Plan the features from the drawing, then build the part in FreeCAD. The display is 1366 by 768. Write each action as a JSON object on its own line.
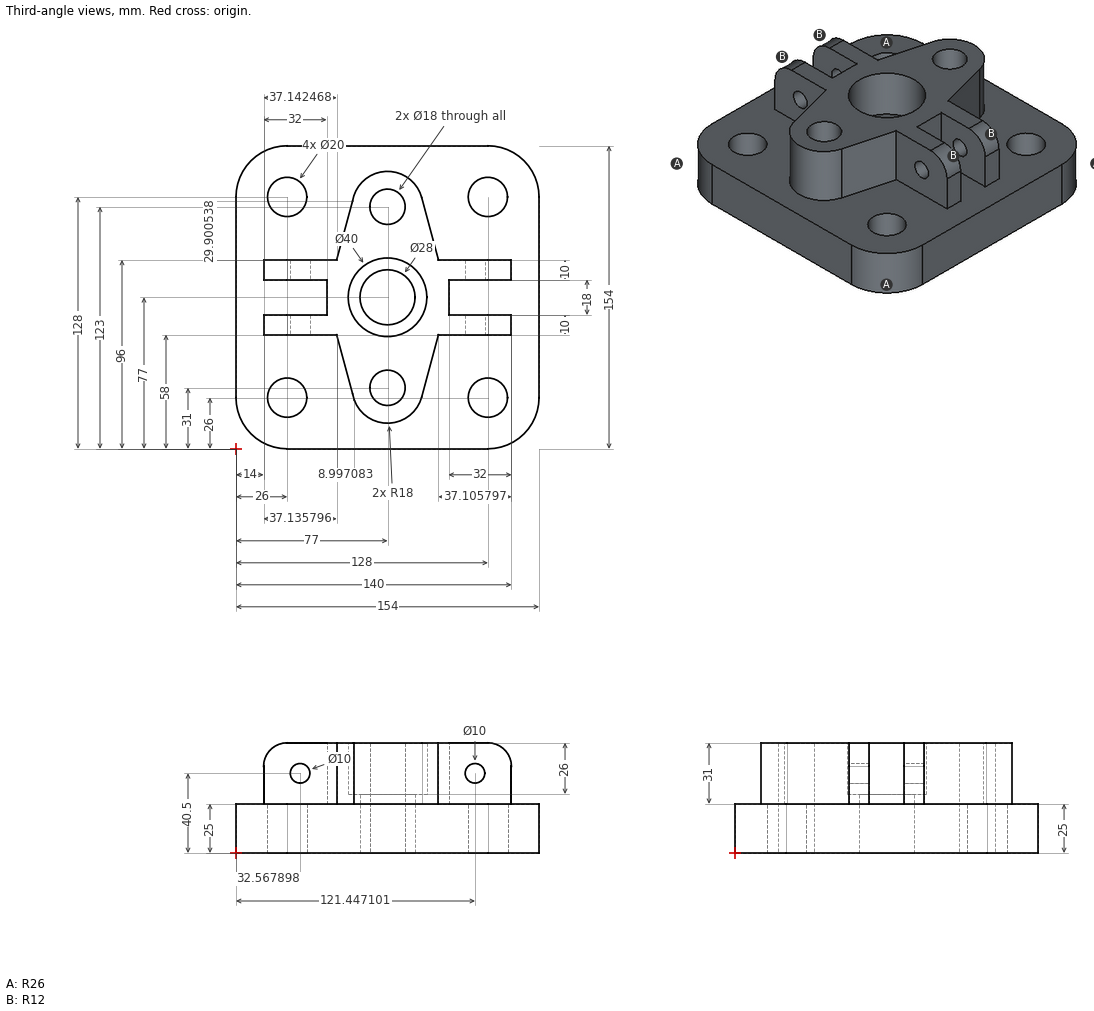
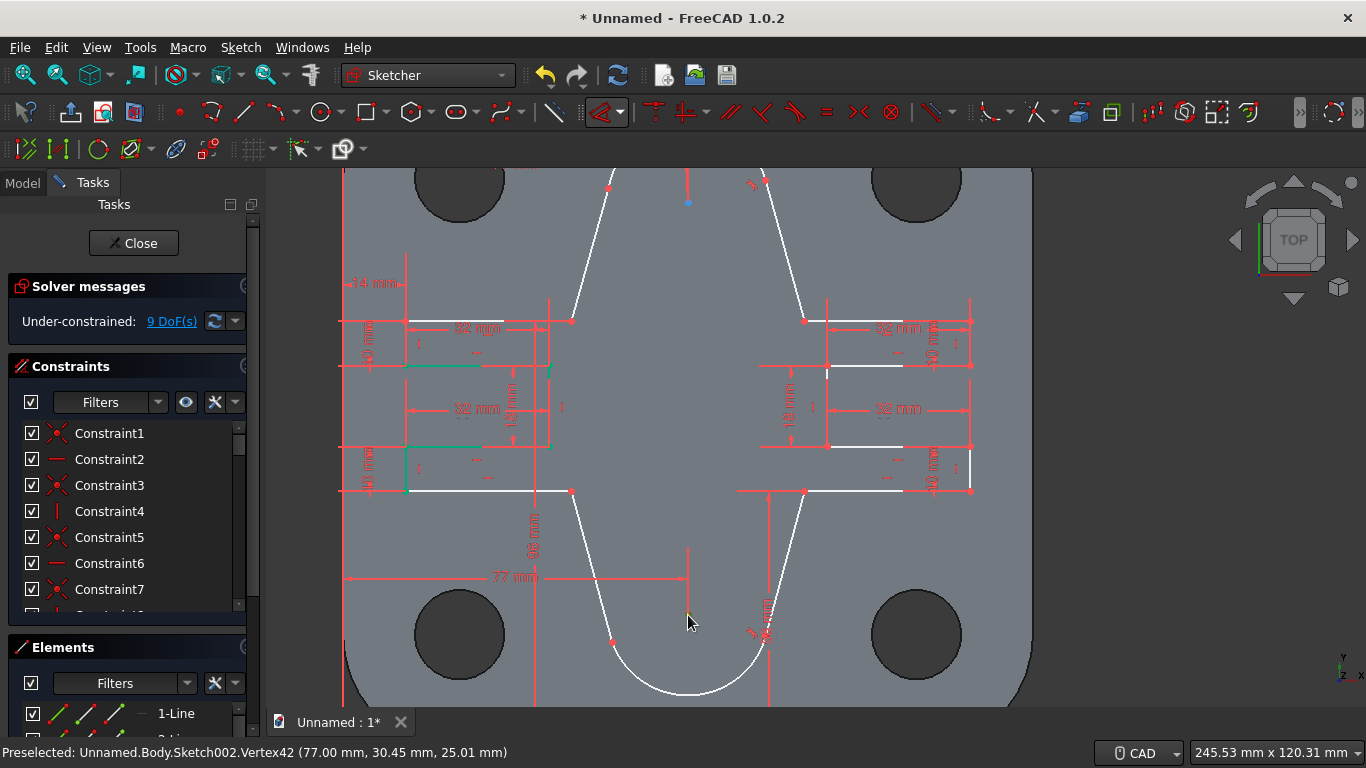
{"action": "key", "text": "i"}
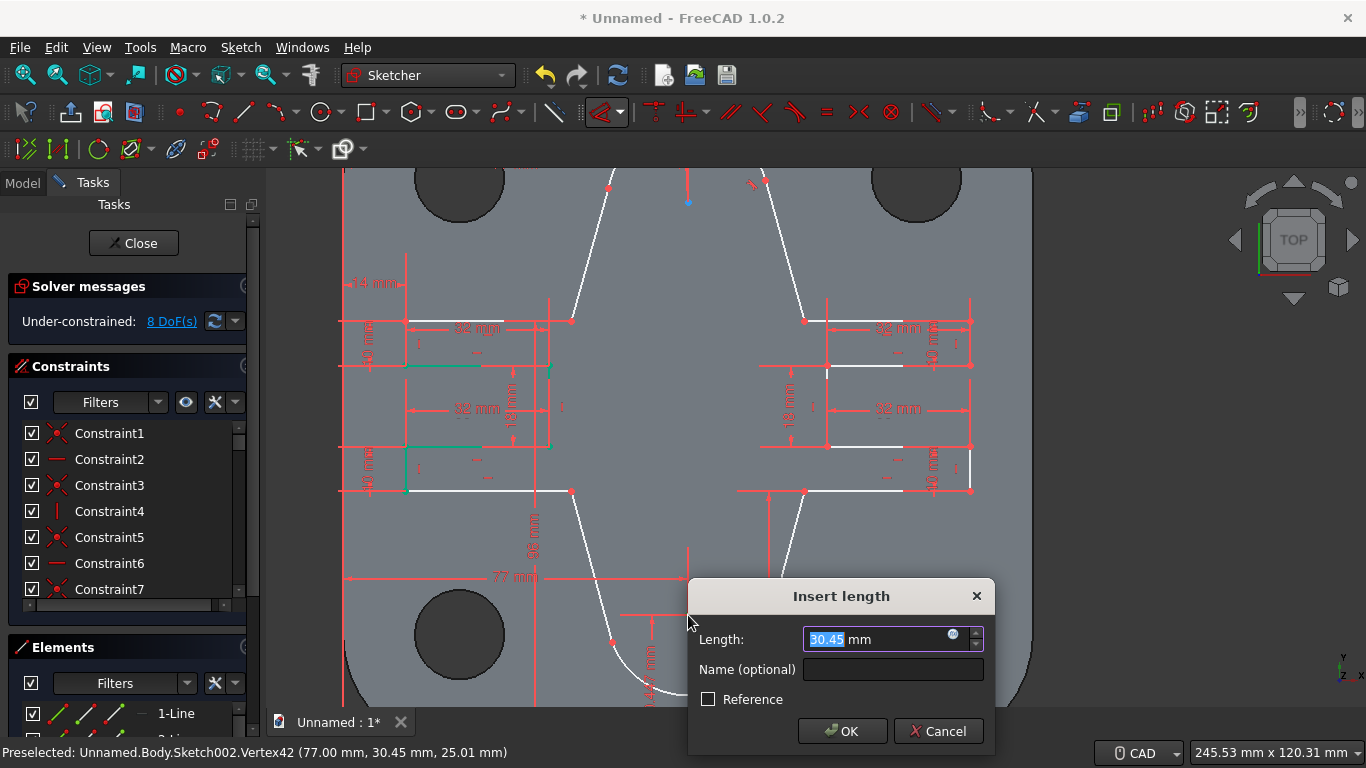
{"action": "type", "text": "31"}
{"action": "key", "text": "Return"}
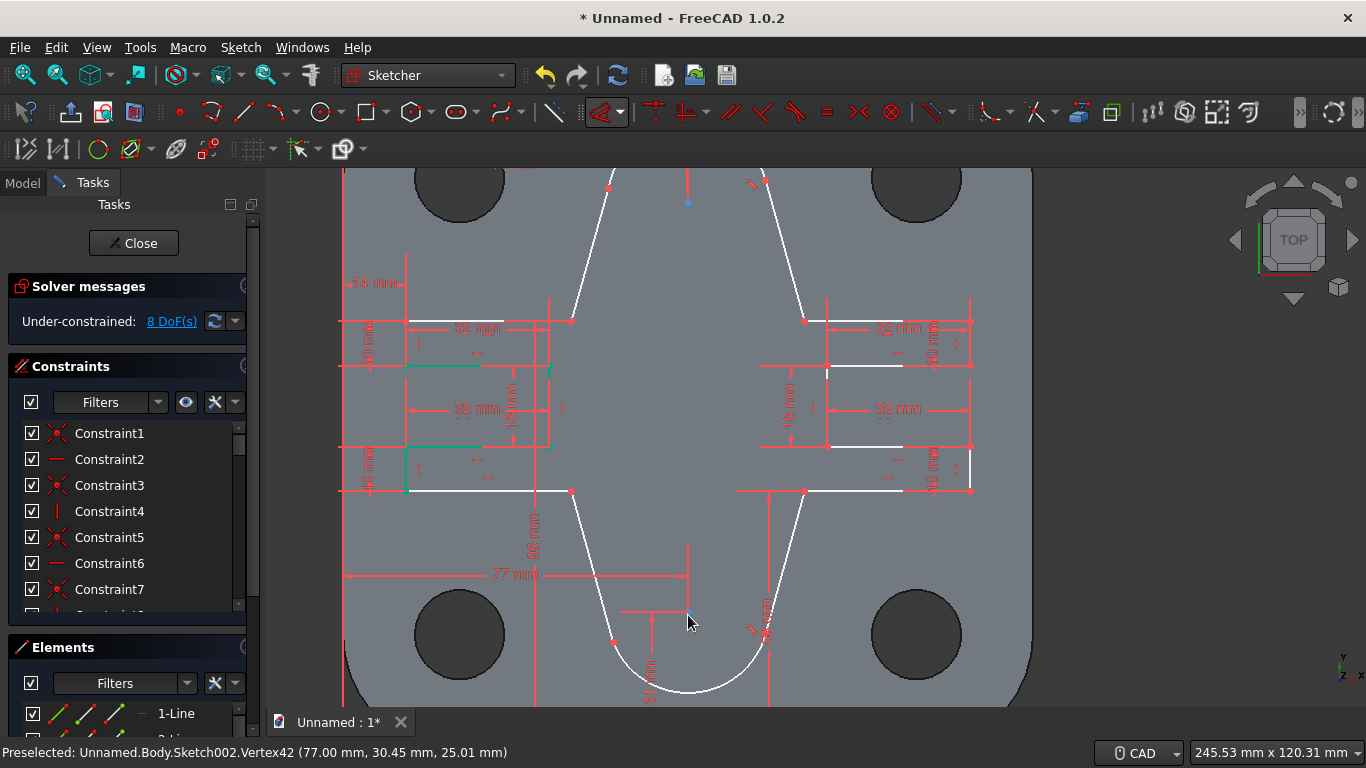
{"action": "left_click", "coordinate": [970, 491]}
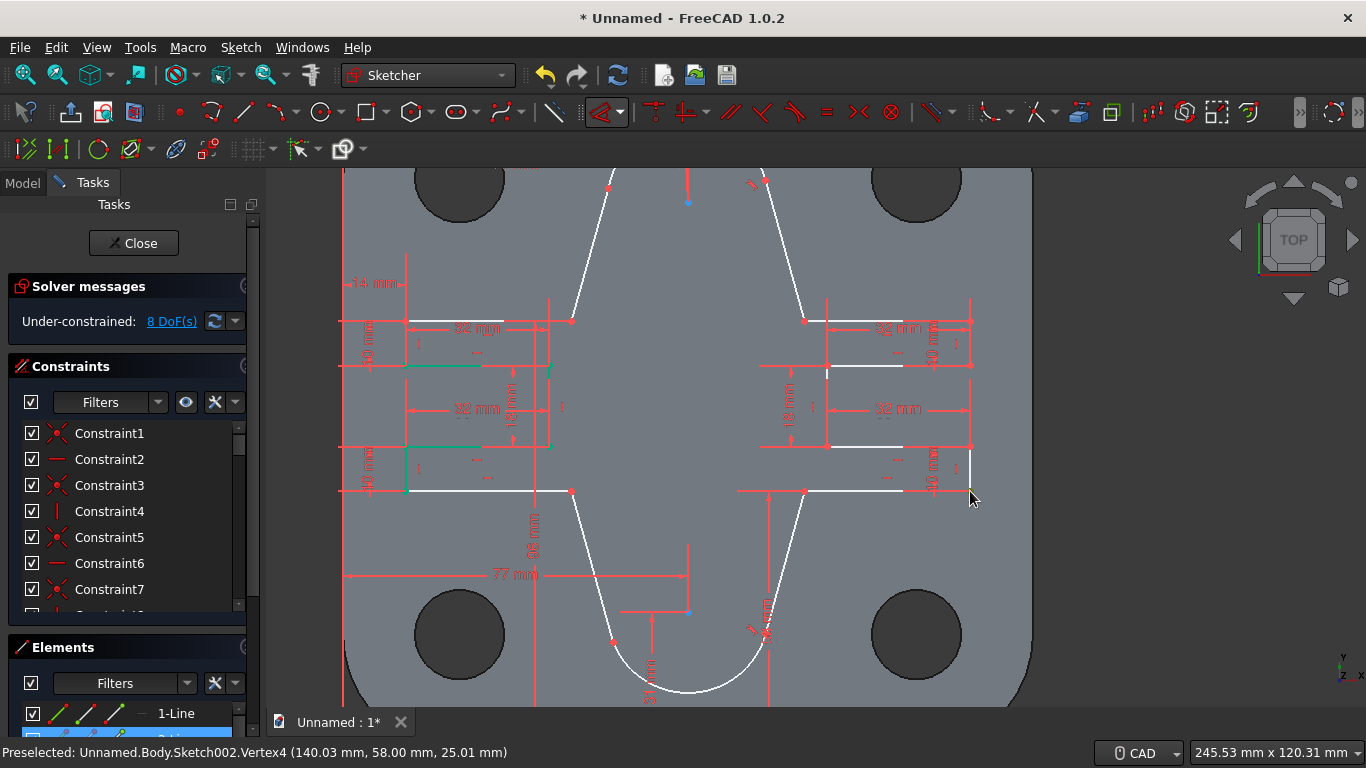
{"action": "left_click", "coordinate": [622, 112]}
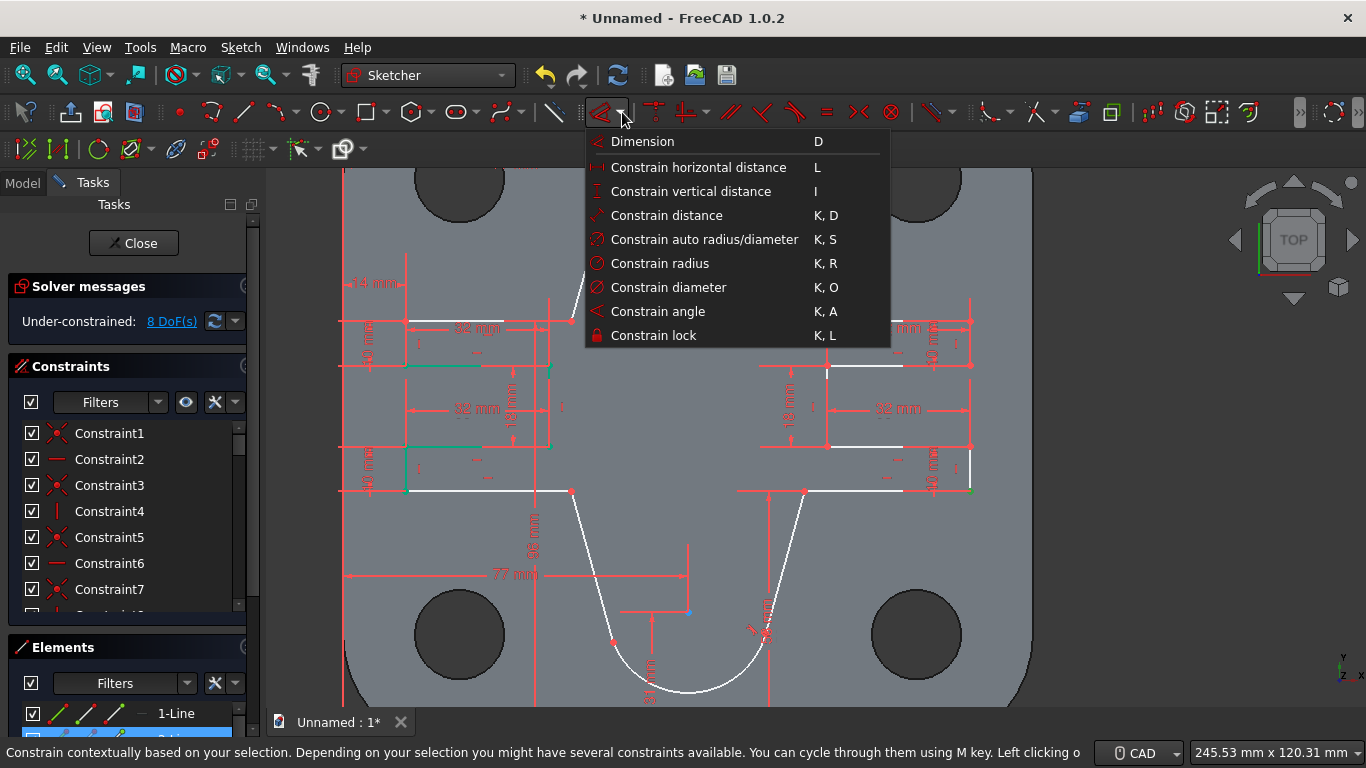
{"action": "left_click", "coordinate": [738, 167]}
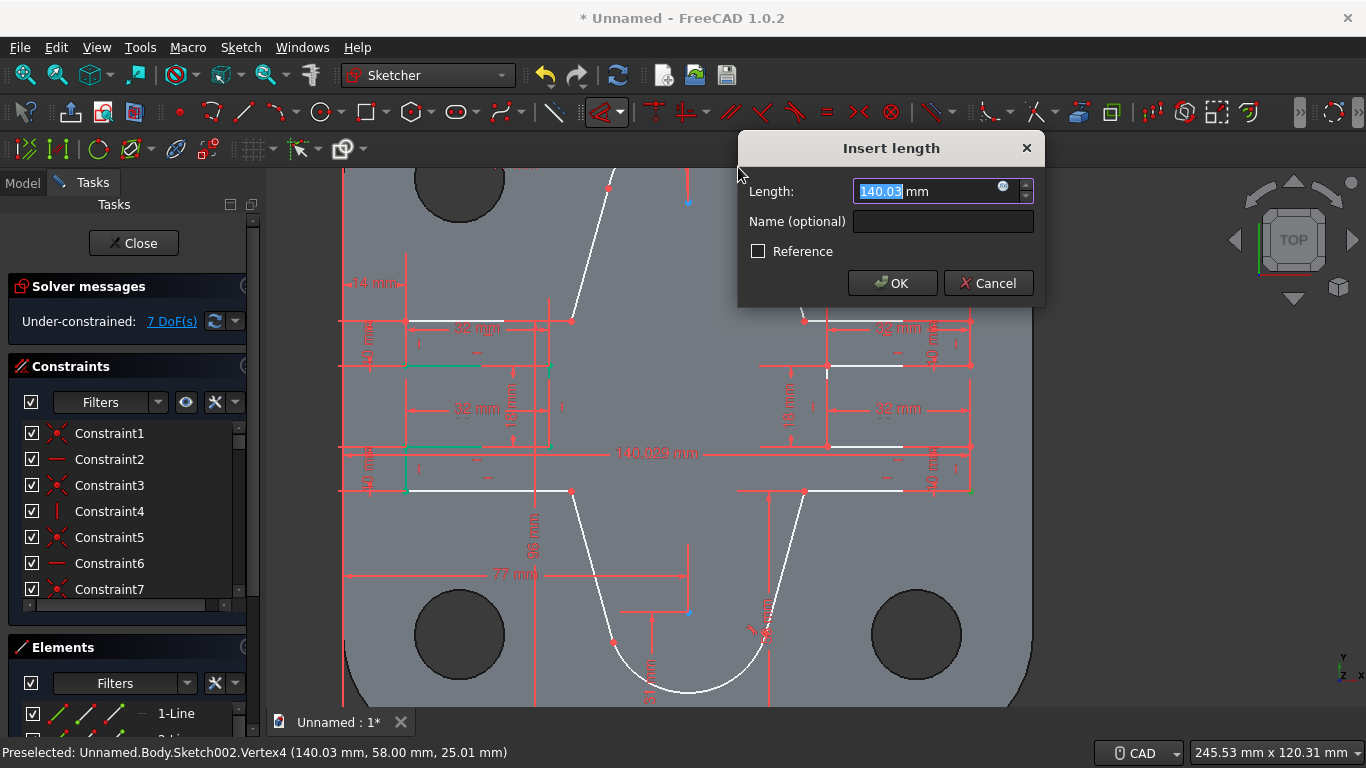
{"action": "type", "text": "140"}
{"action": "key", "text": "Return"}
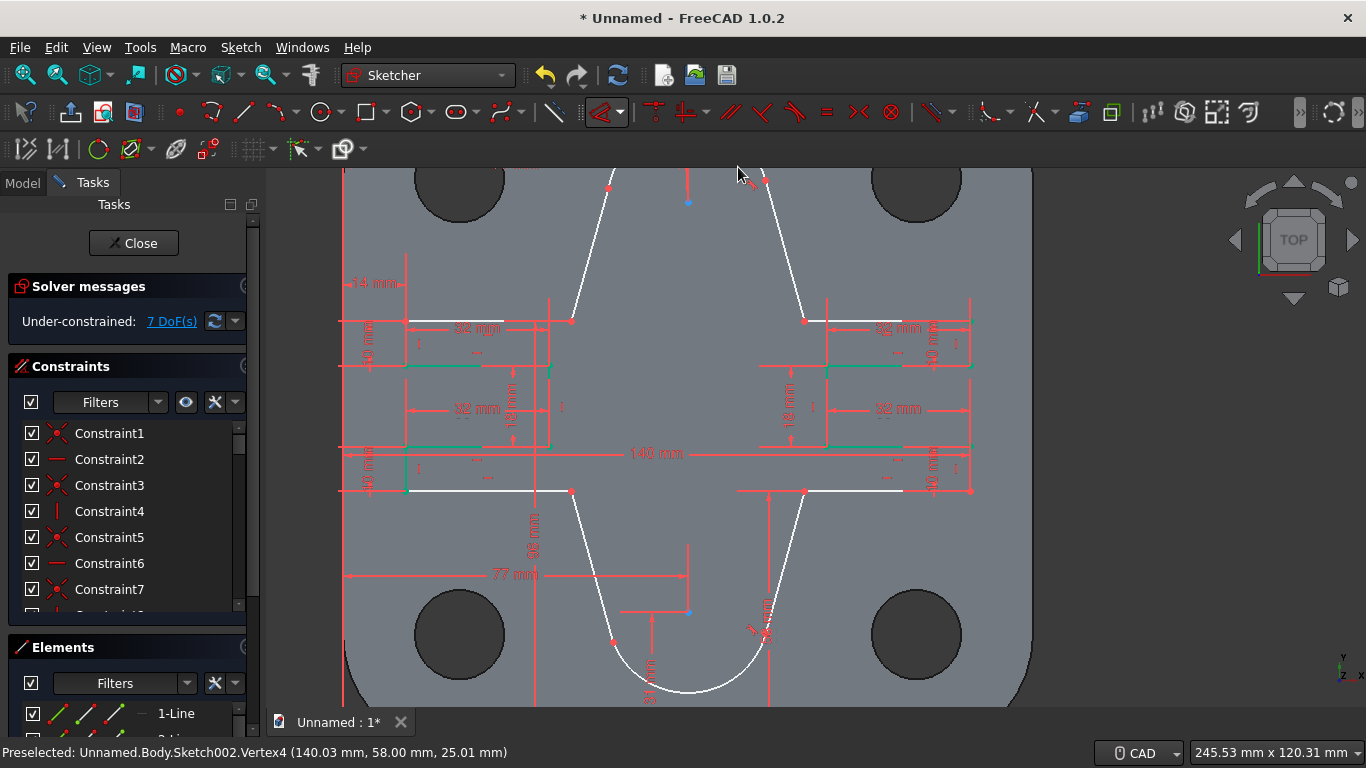
{"action": "left_click", "coordinate": [688, 202]}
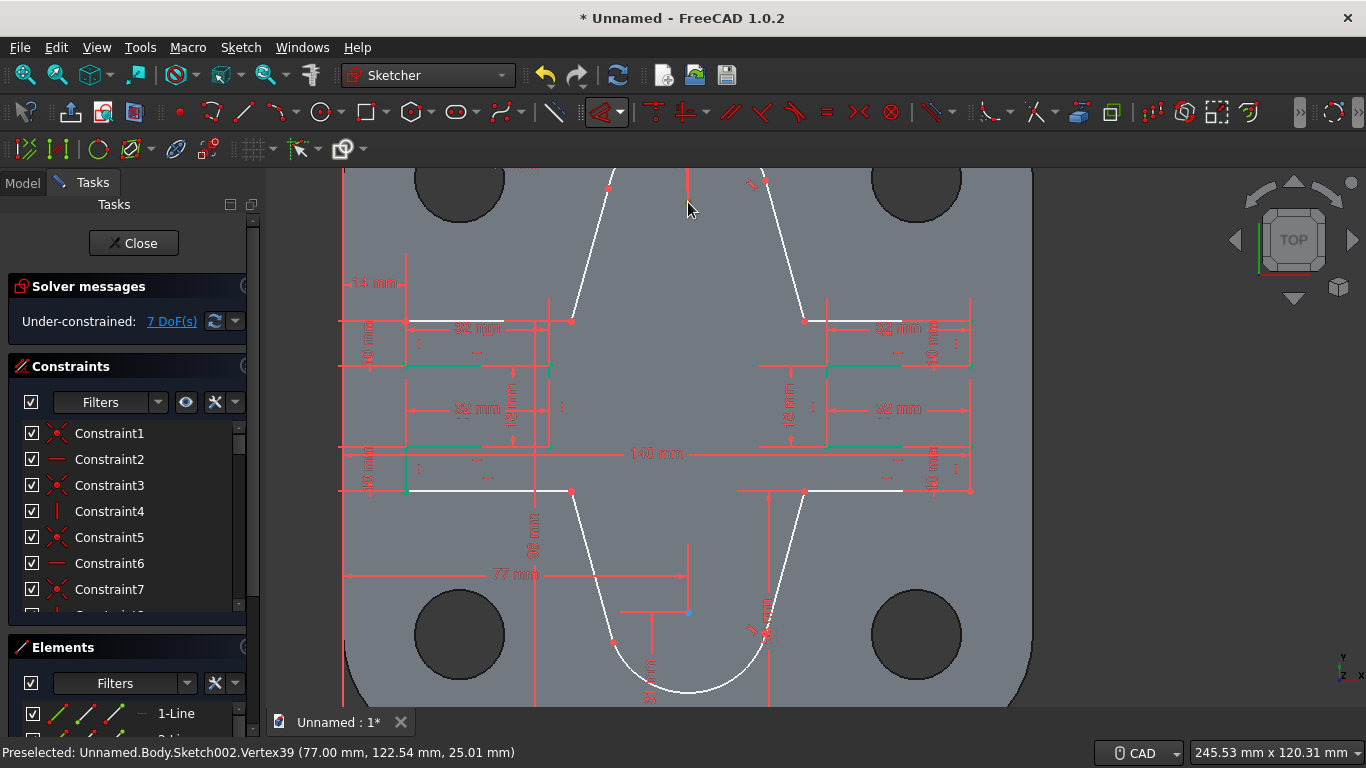
{"action": "left_click", "coordinate": [622, 112]}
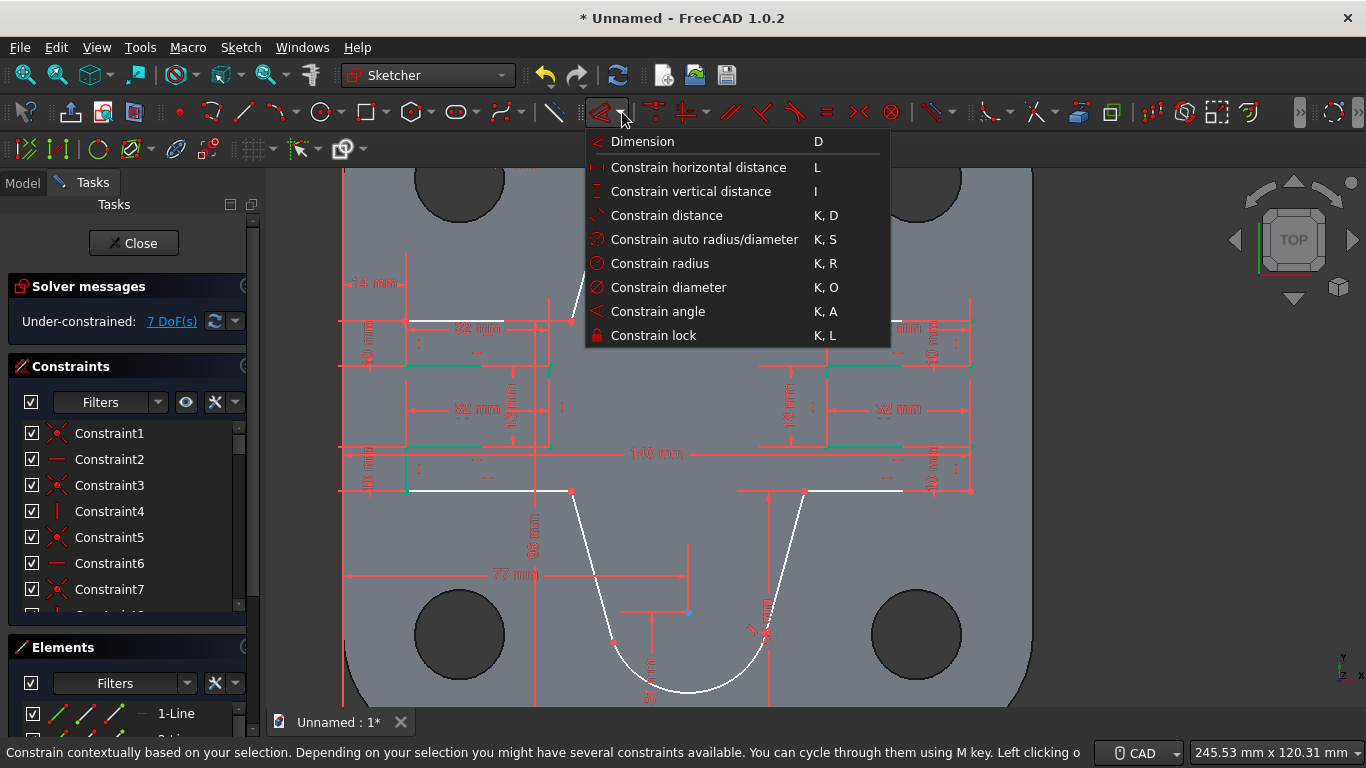
{"action": "left_click", "coordinate": [738, 191]}